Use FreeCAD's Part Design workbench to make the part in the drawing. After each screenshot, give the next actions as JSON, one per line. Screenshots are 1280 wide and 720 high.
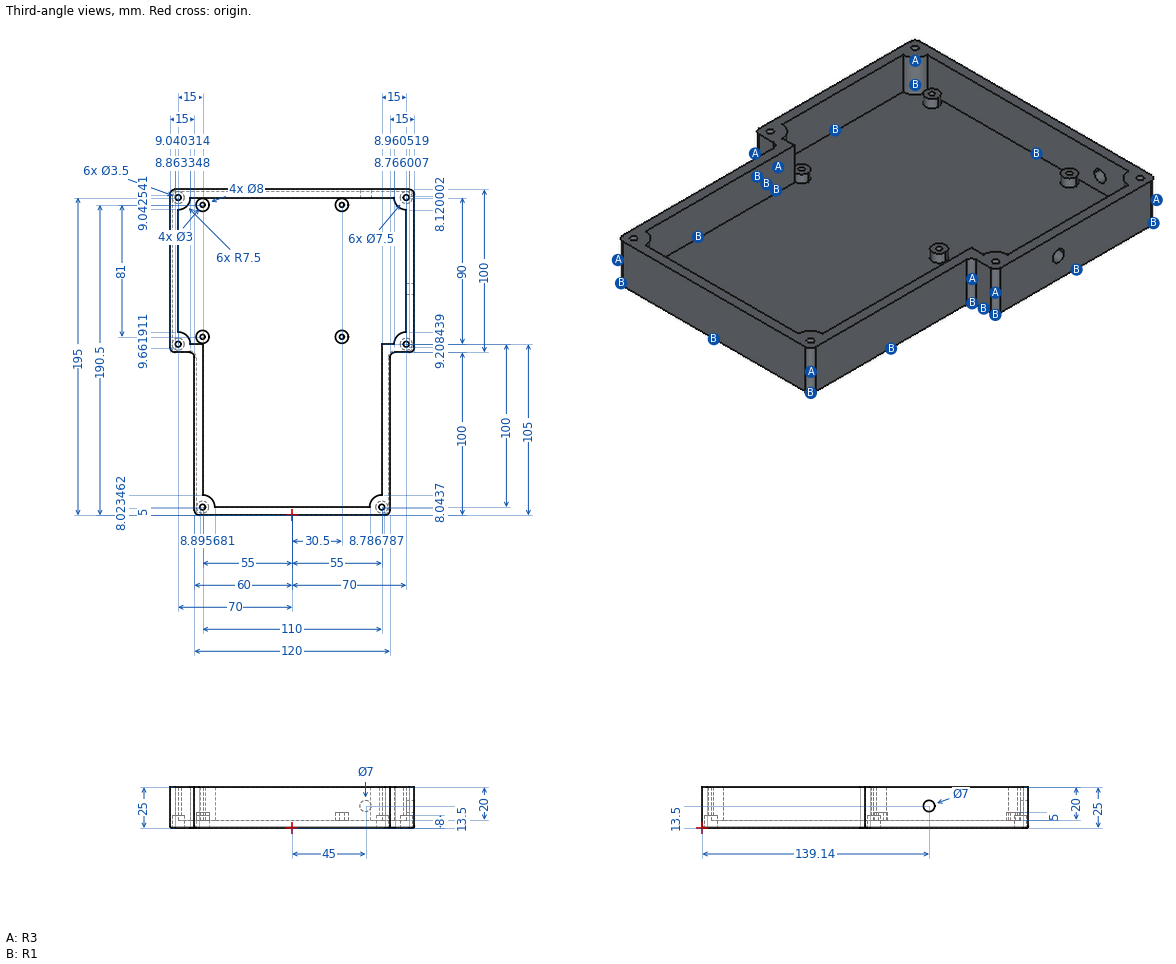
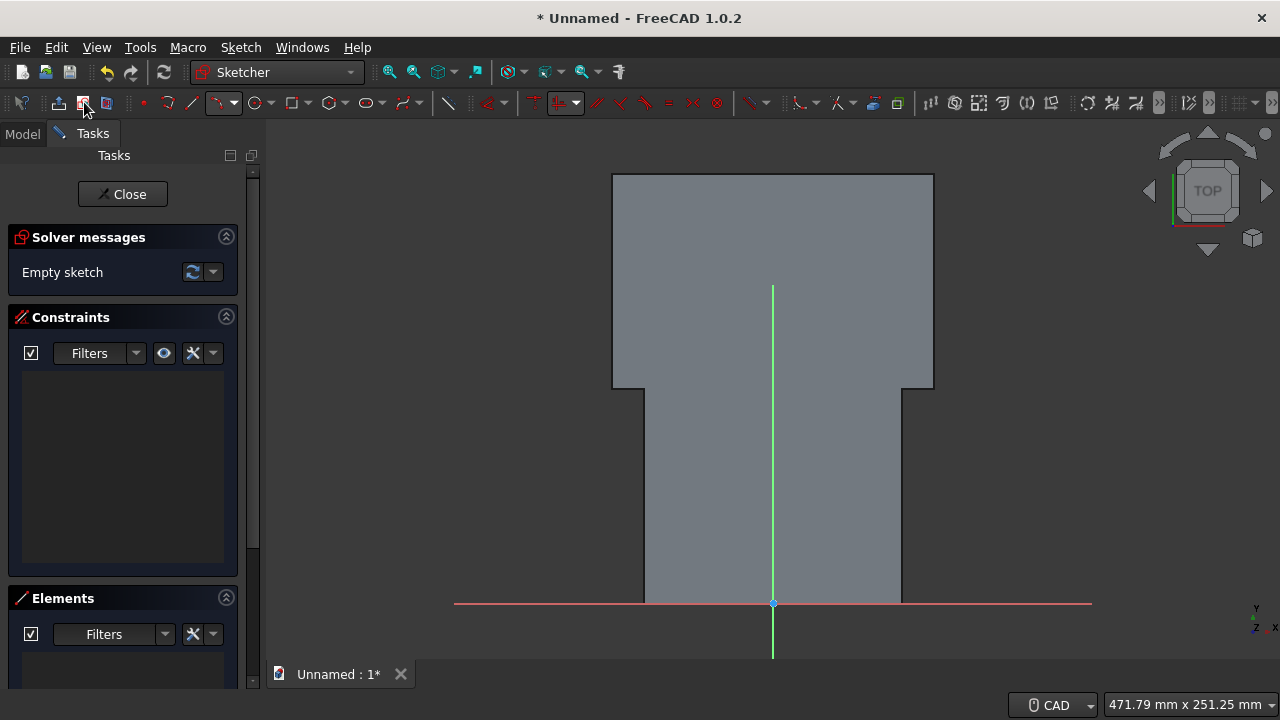
{"action": "left_click", "coordinate": [168, 104]}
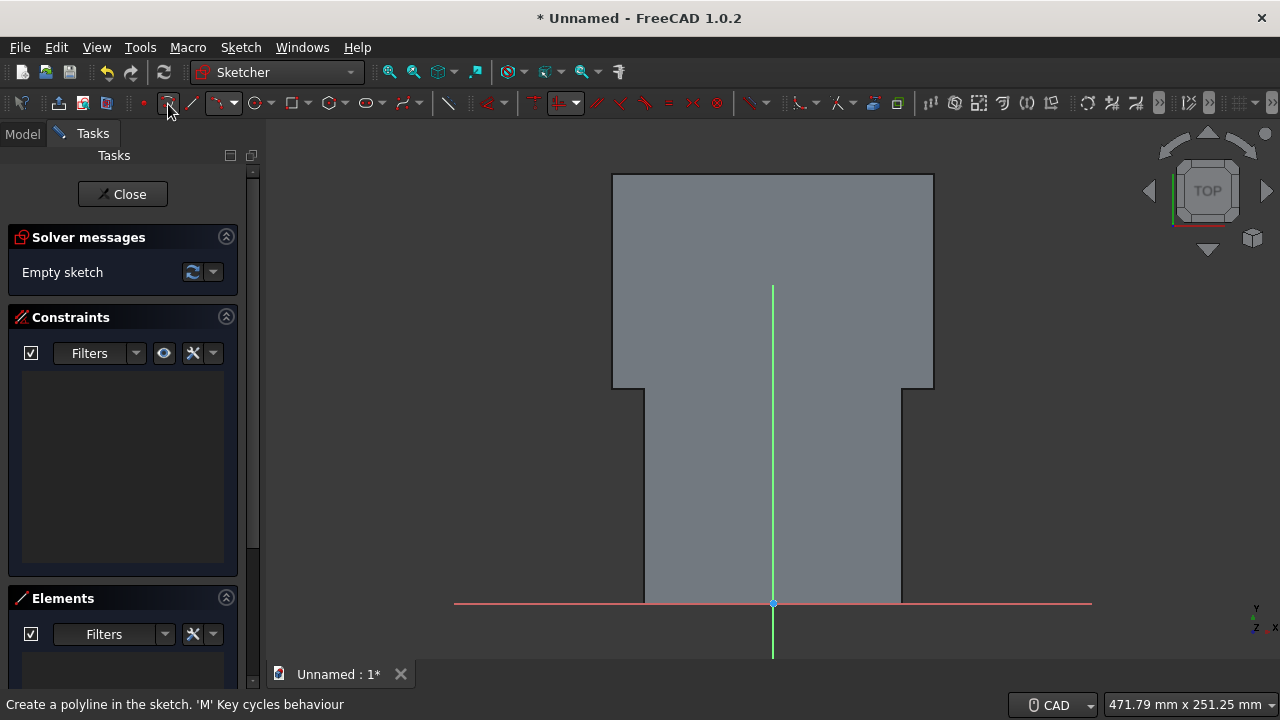
{"action": "scroll", "coordinate": [655, 593], "scroll_direction": "up", "scroll_amount": 2}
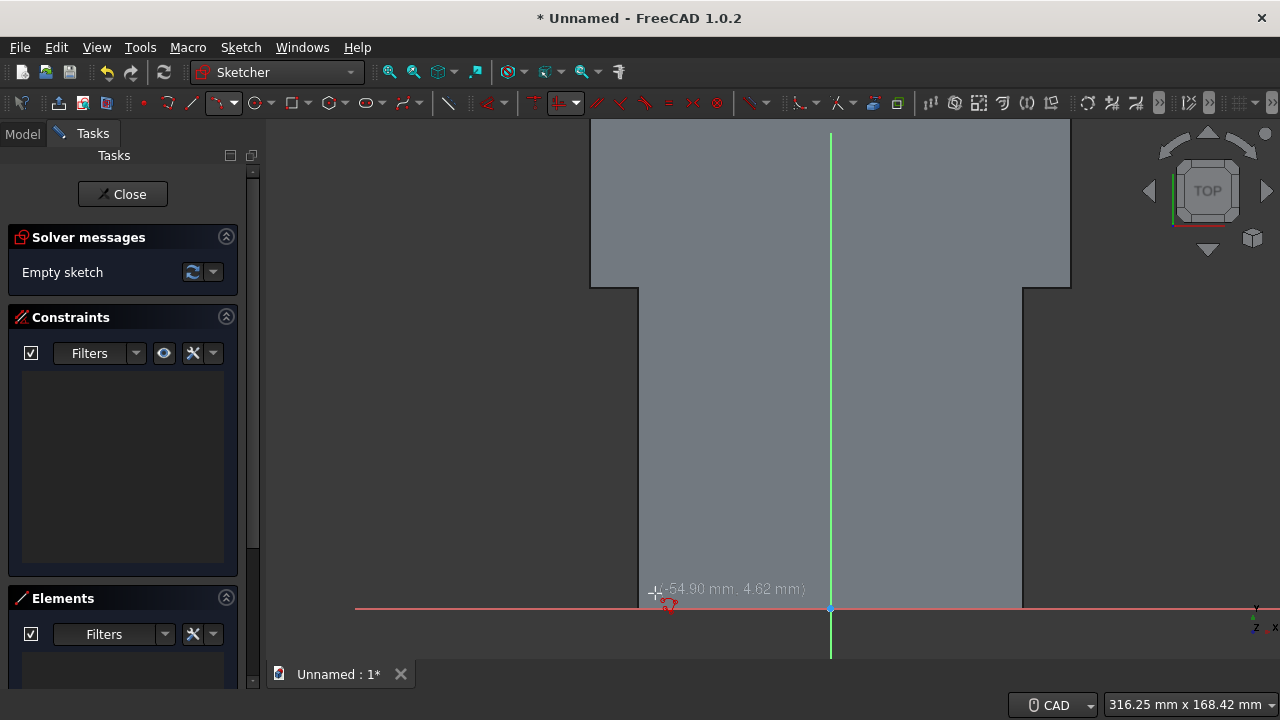
{"action": "left_click", "coordinate": [654, 593]}
{"action": "left_click", "coordinate": [1007, 593]}
{"action": "left_click", "coordinate": [1007, 272]}
{"action": "left_click", "coordinate": [1055, 272]}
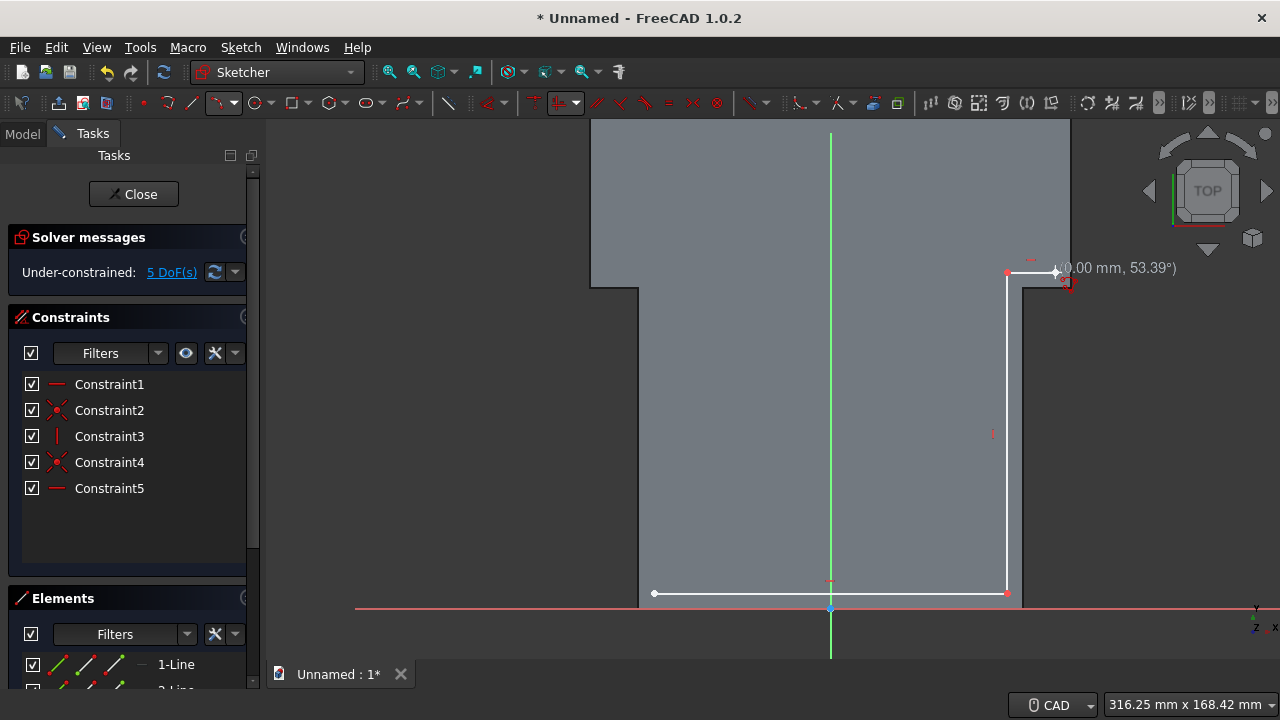
{"action": "scroll", "coordinate": [551, 502], "scroll_direction": "down", "scroll_amount": 3}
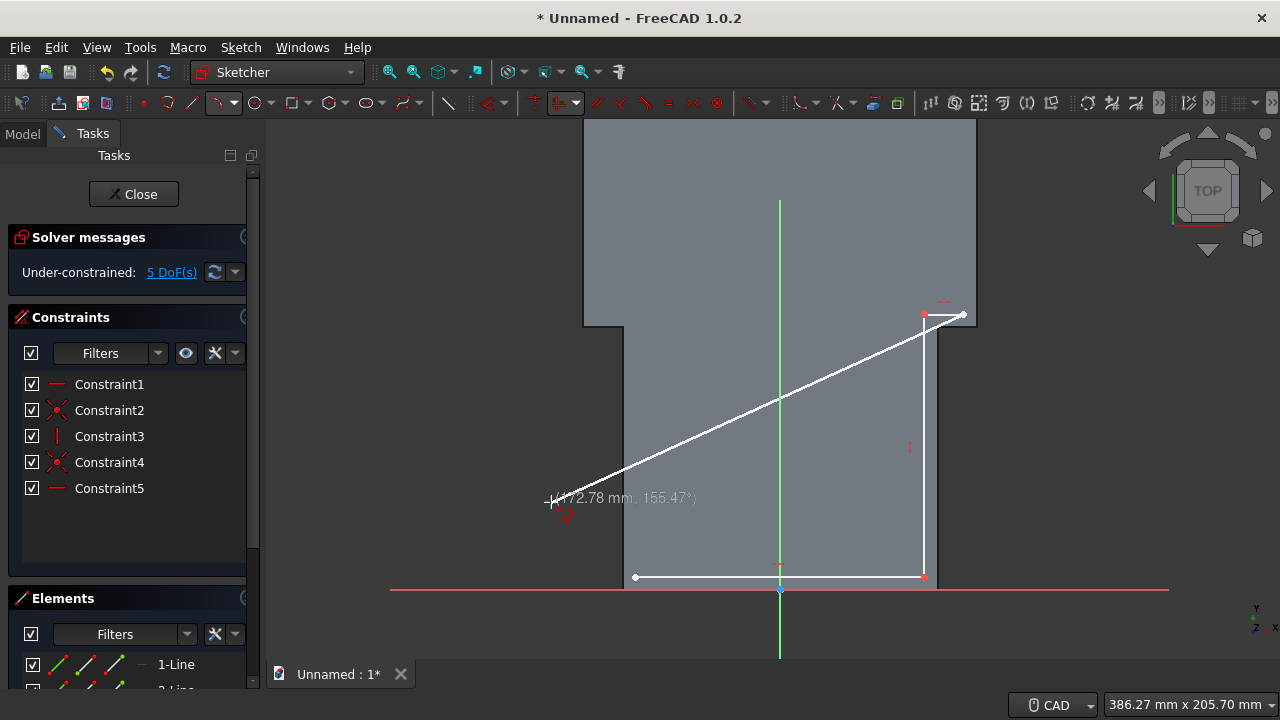
{"action": "left_click", "coordinate": [828, 218]}
{"action": "left_click", "coordinate": [582, 218]}
{"action": "left_click", "coordinate": [582, 376]}
{"action": "left_click", "coordinate": [608, 376]}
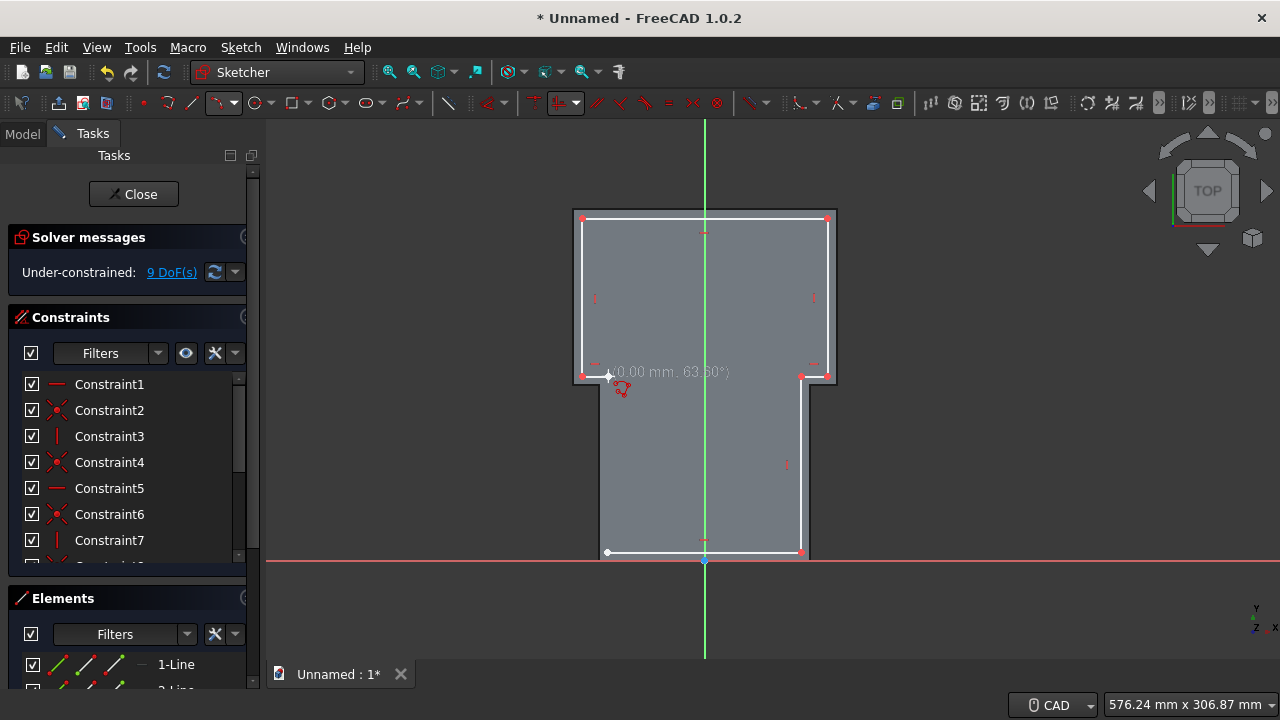
{"action": "scroll", "coordinate": [608, 552], "scroll_direction": "up", "scroll_amount": 3}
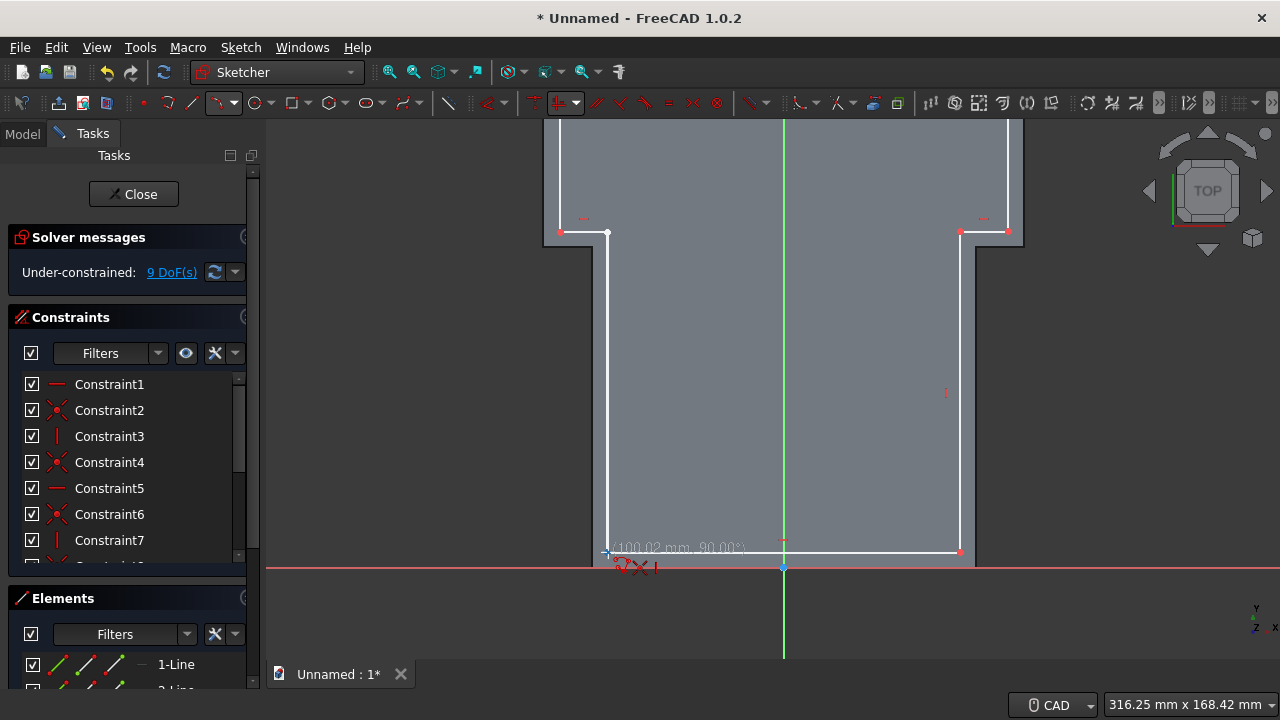
{"action": "left_click", "coordinate": [607, 553]}
{"action": "key", "text": "Escape"}
{"action": "key", "text": "Escape"}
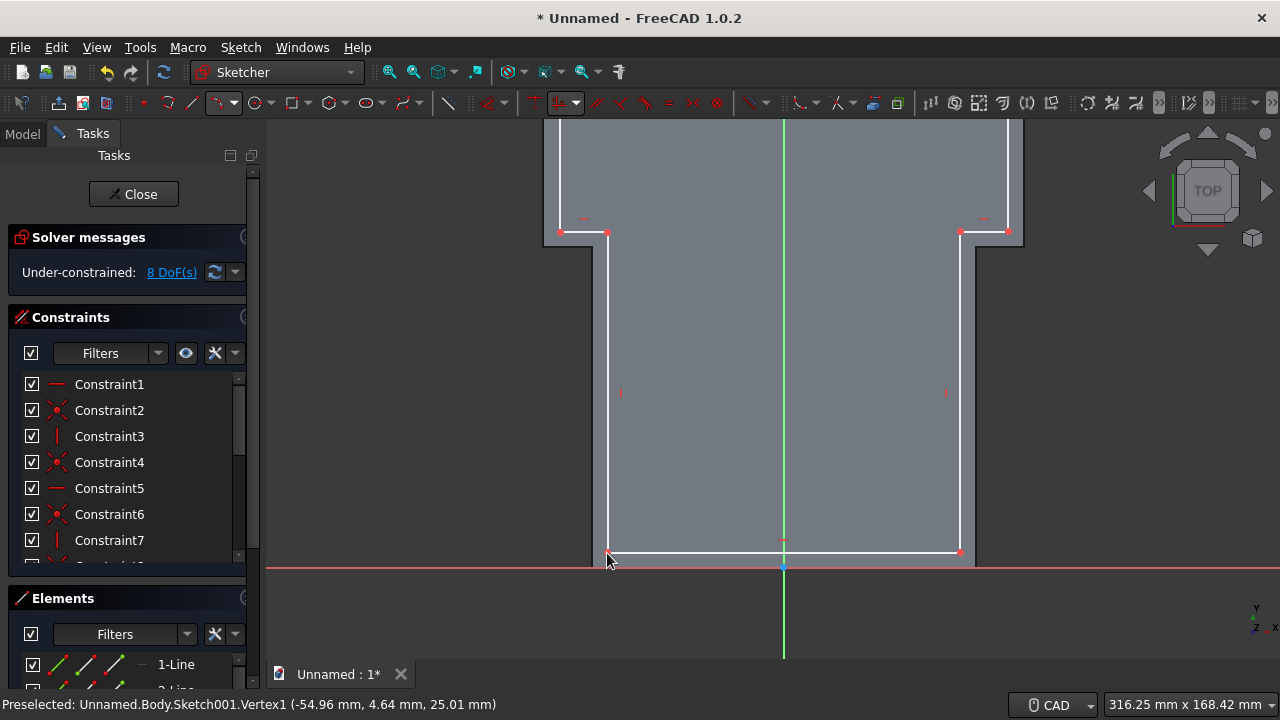
{"action": "key", "text": "d"}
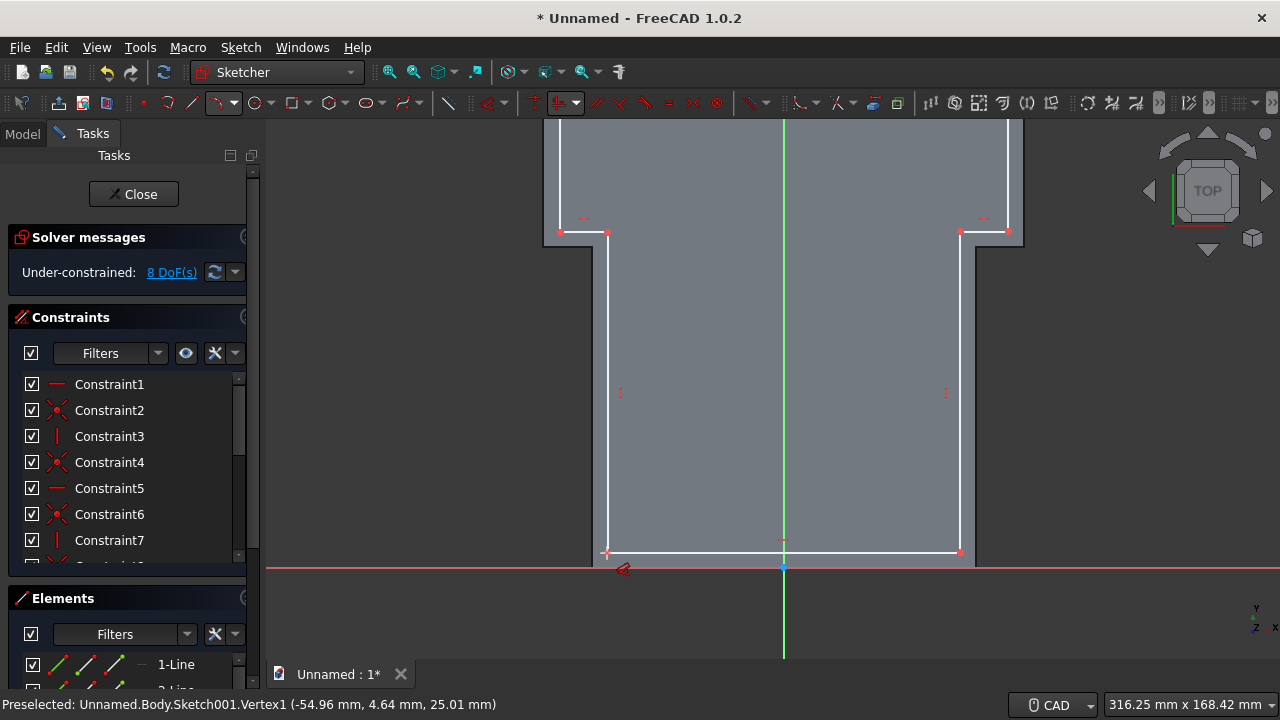
{"action": "left_click", "coordinate": [974, 232]}
{"action": "left_click", "coordinate": [984, 198]}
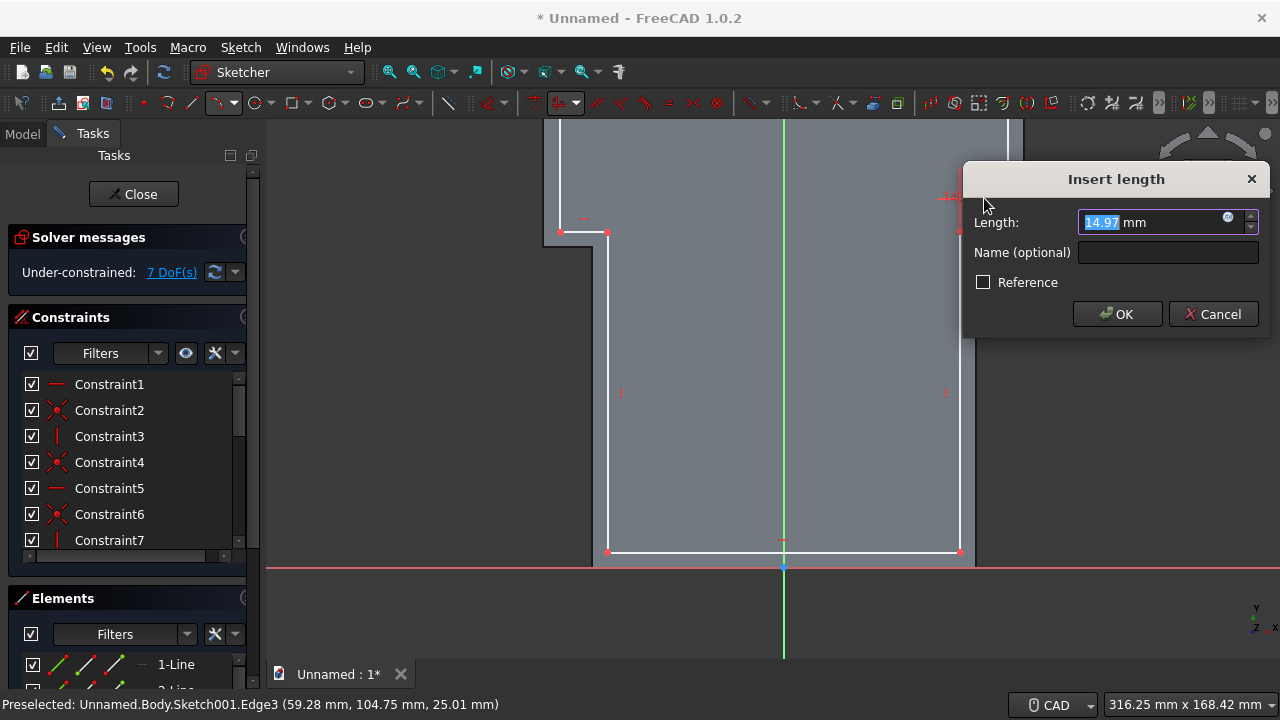
{"action": "type", "text": "15"}
{"action": "key", "text": "Return"}